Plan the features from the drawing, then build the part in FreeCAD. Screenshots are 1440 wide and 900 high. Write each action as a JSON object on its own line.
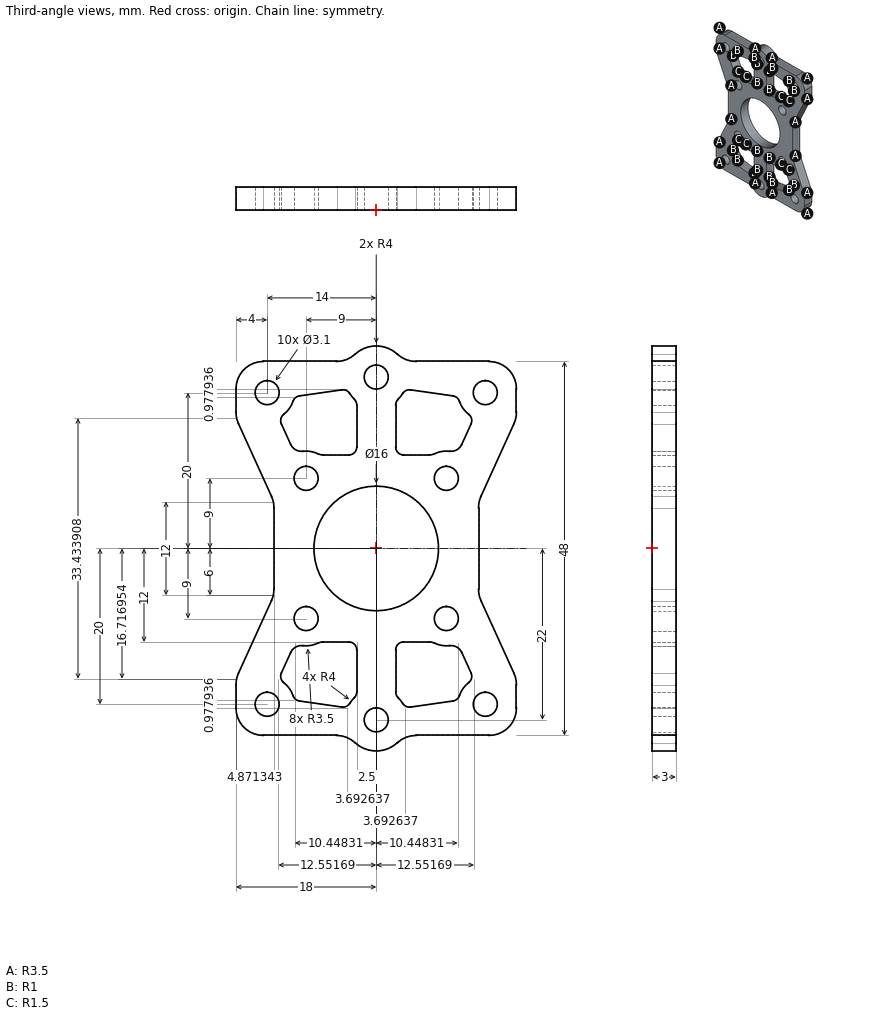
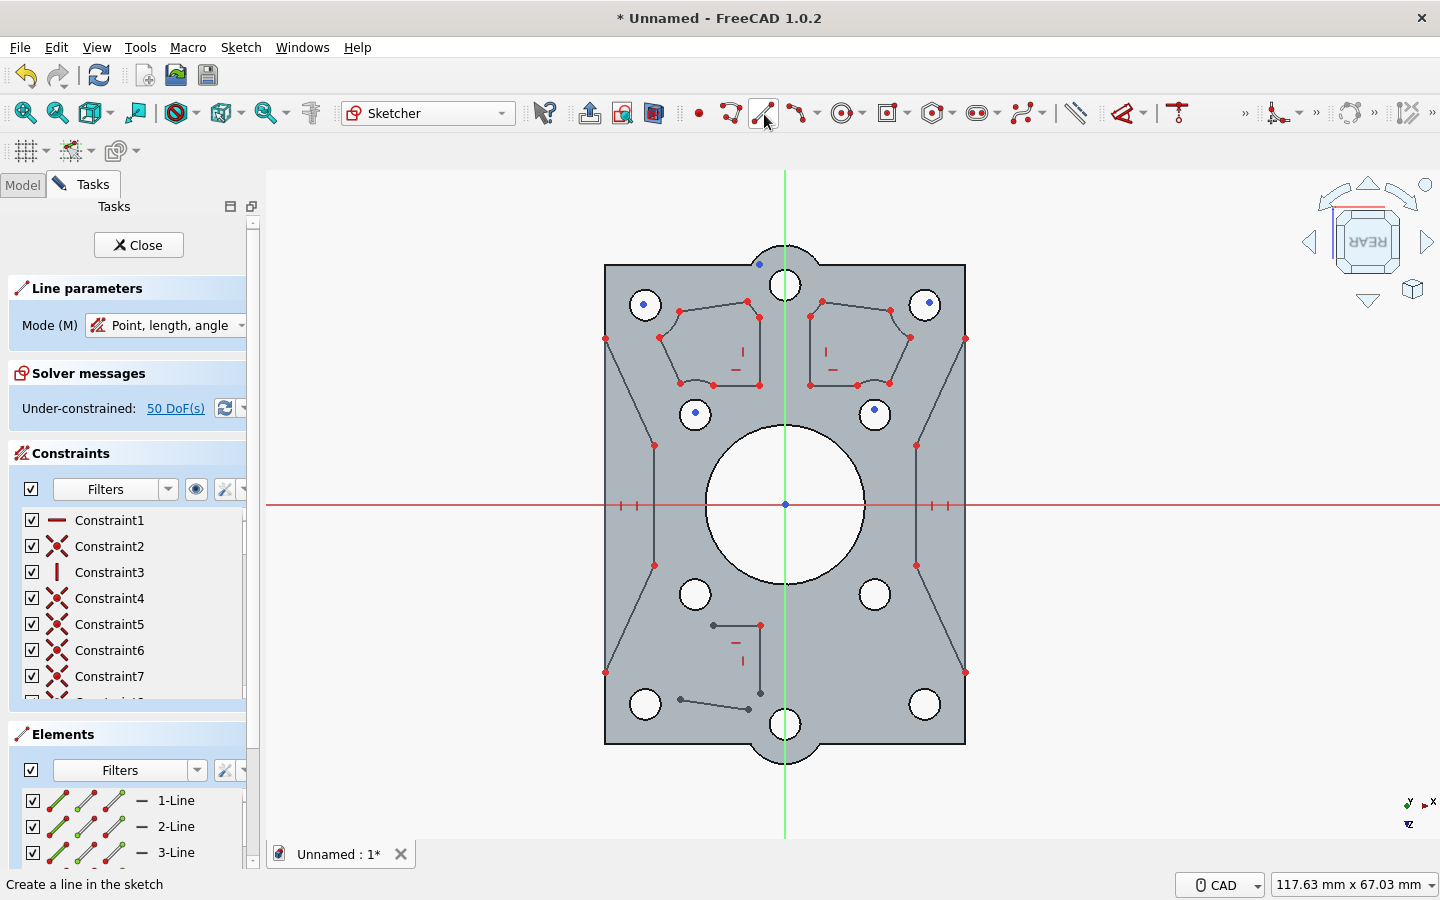
{"action": "left_click", "coordinate": [681, 626]}
{"action": "left_click", "coordinate": [660, 673]}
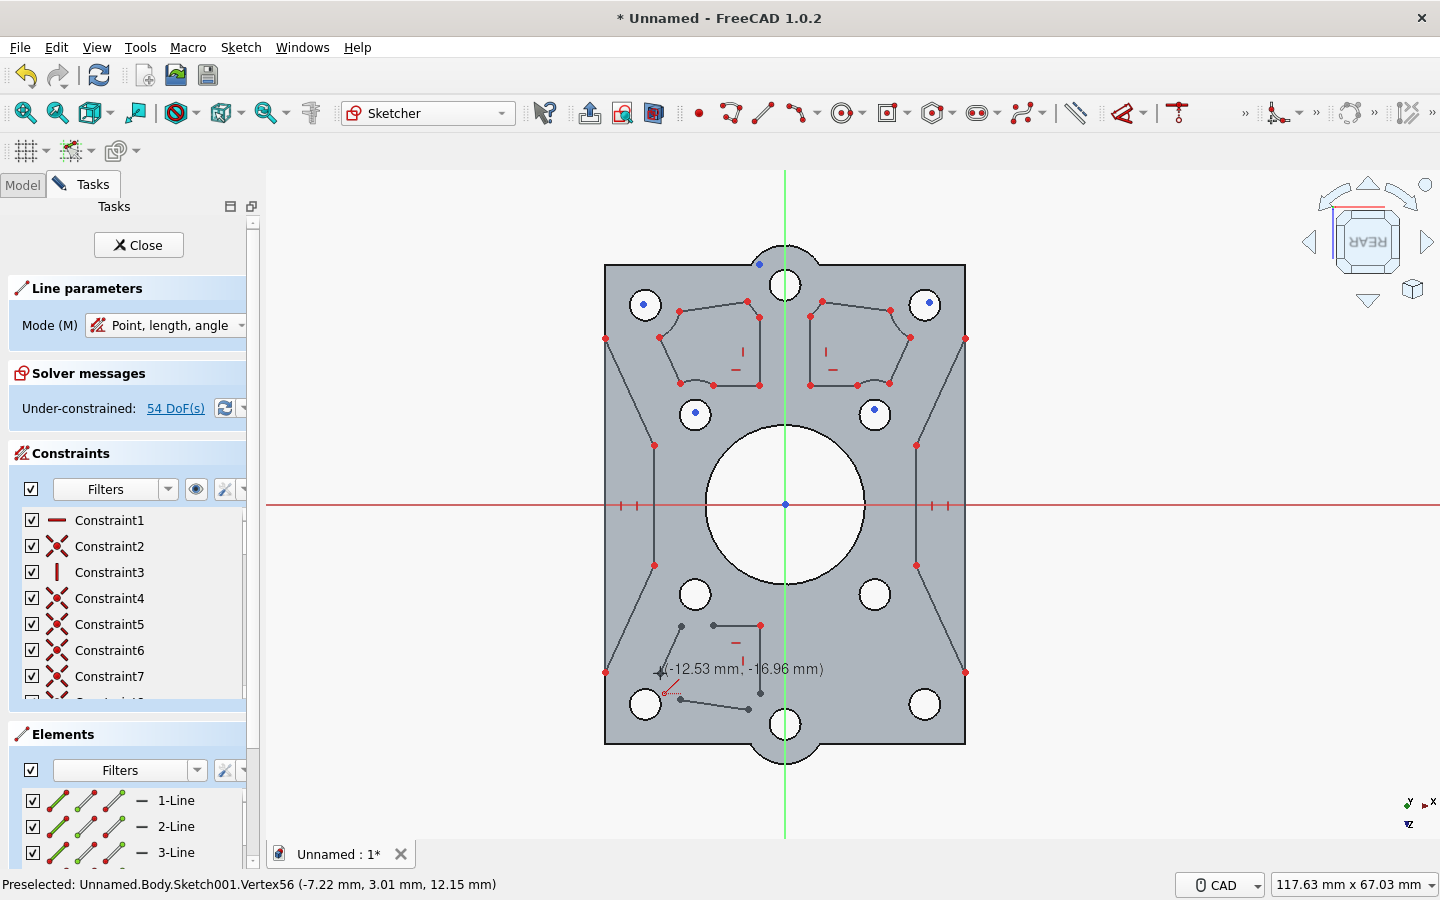
{"action": "left_click", "coordinate": [796, 114]}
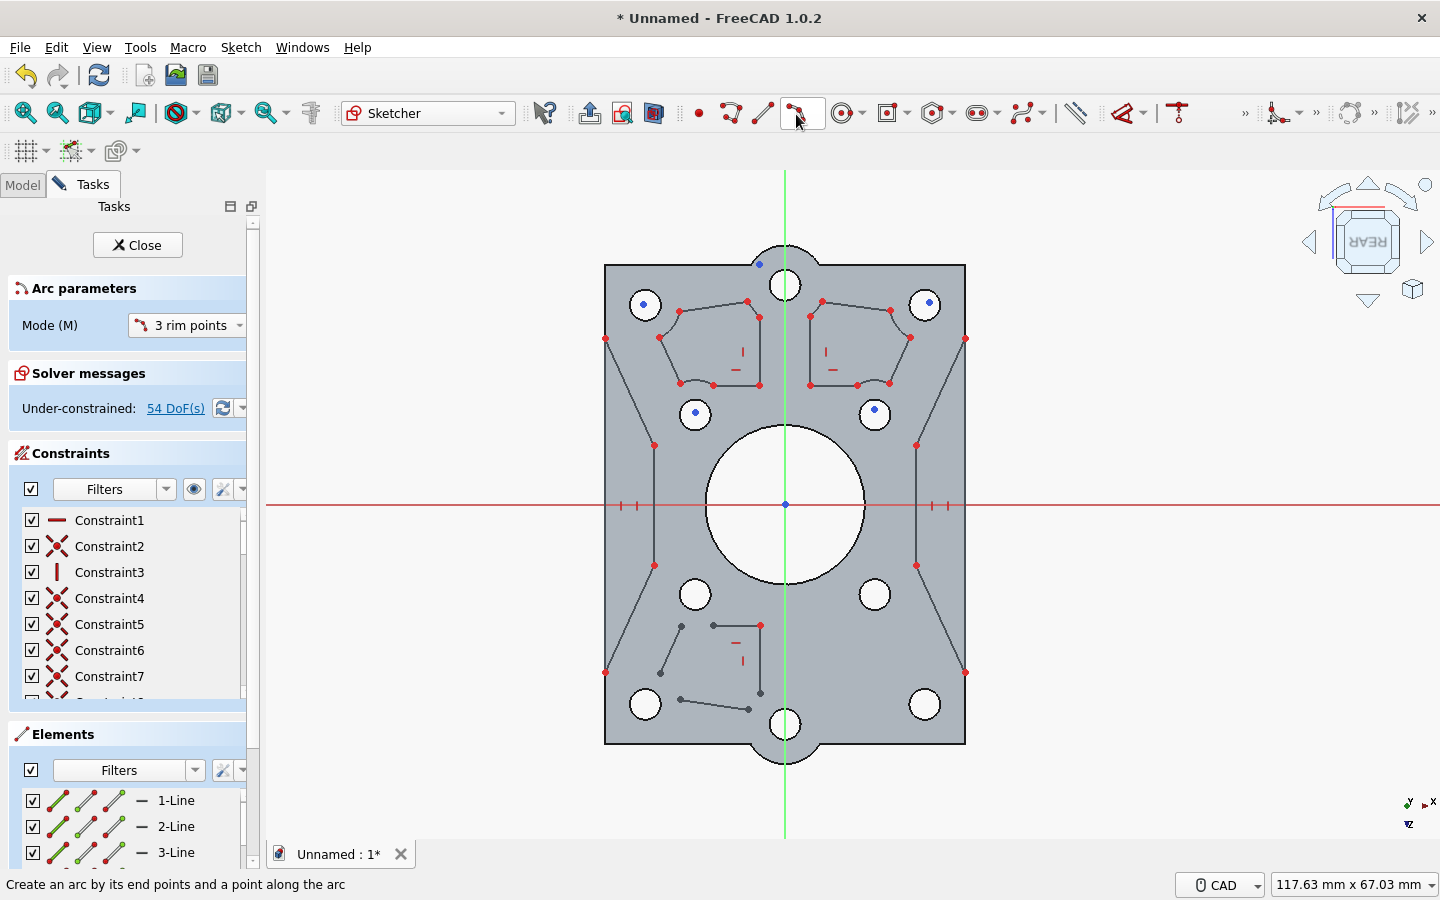
{"action": "left_click", "coordinate": [748, 710]}
{"action": "left_click", "coordinate": [760, 694]}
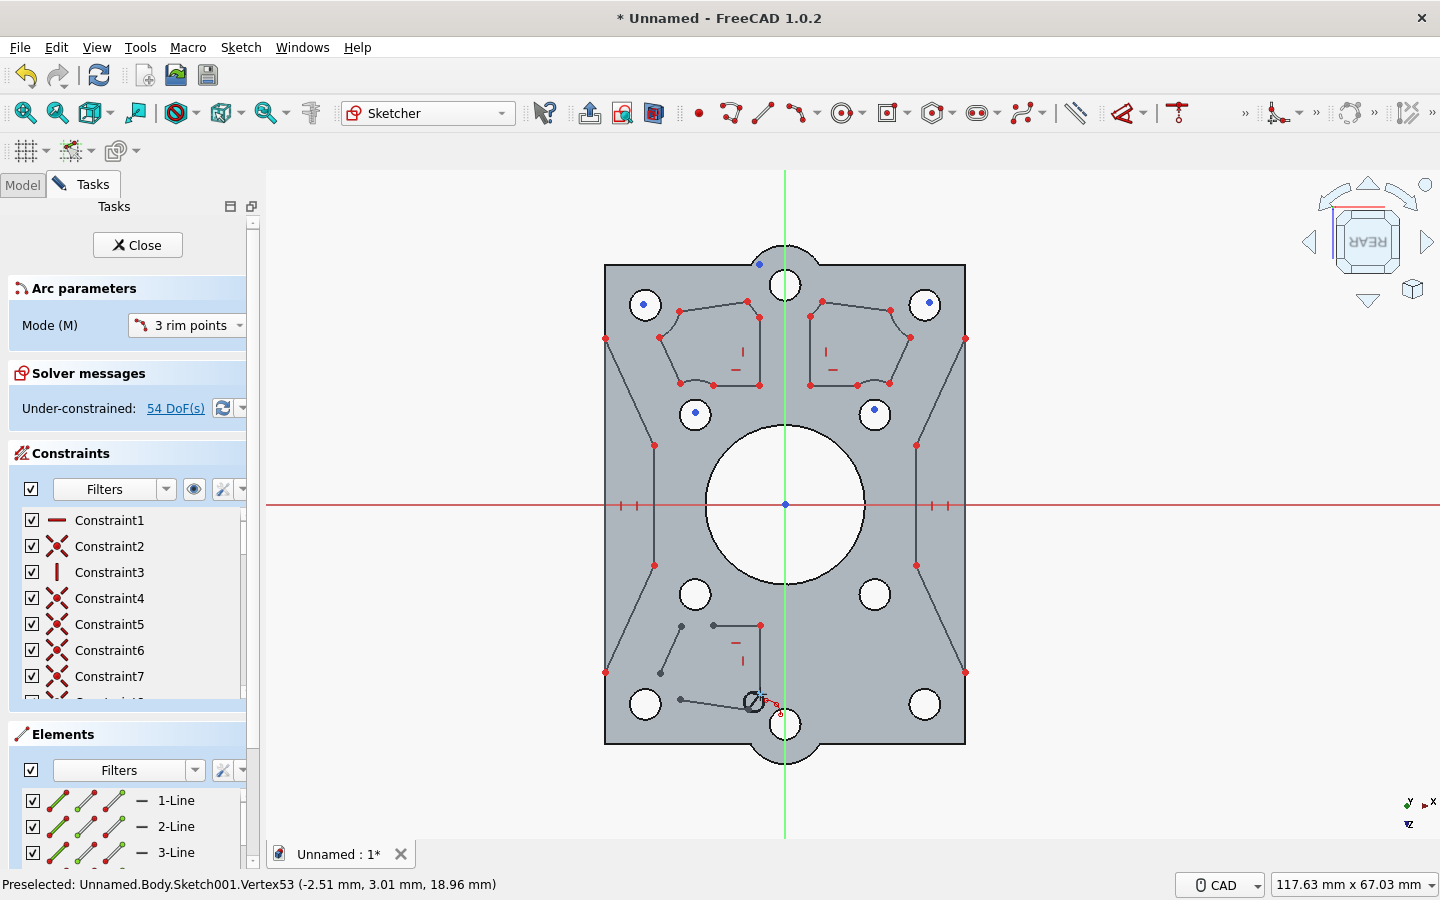
{"action": "scroll", "coordinate": [753, 700], "scroll_direction": "up", "scroll_amount": 13}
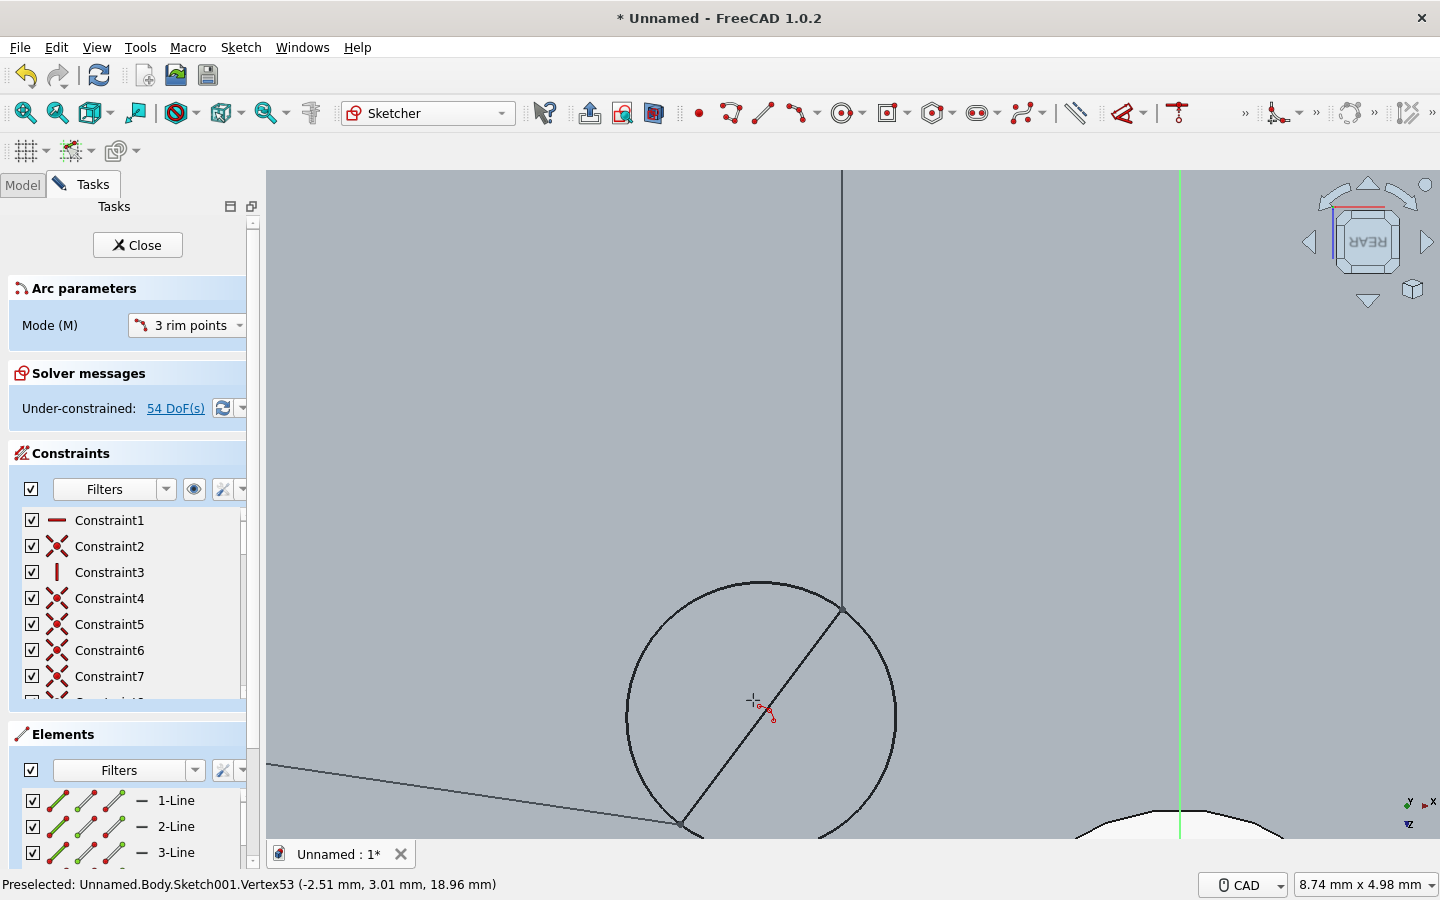
{"action": "left_click", "coordinate": [750, 694]}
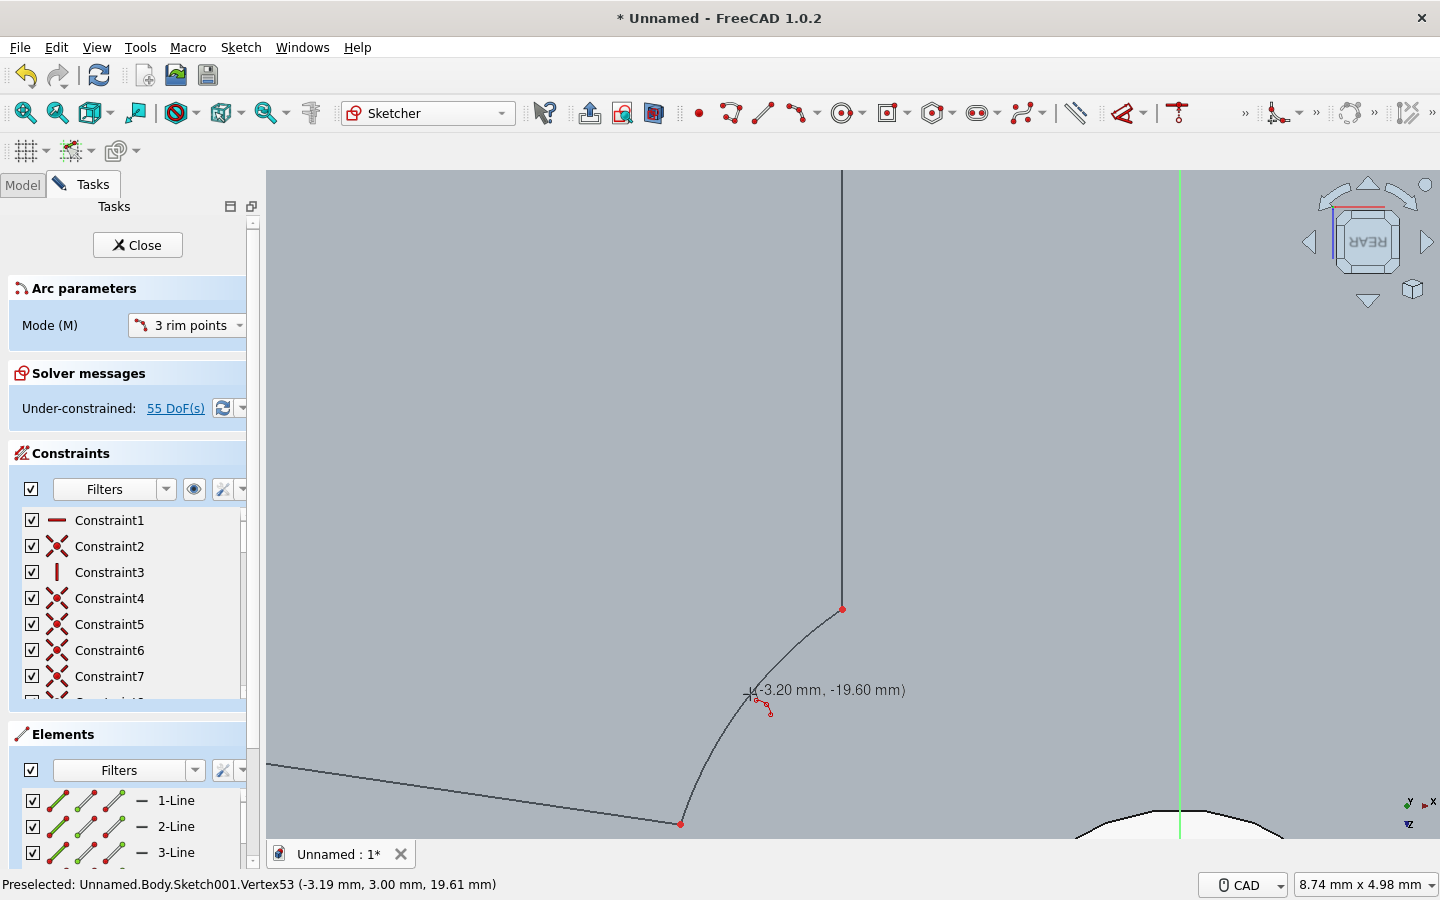
{"action": "scroll", "coordinate": [753, 701], "scroll_direction": "down", "scroll_amount": 13}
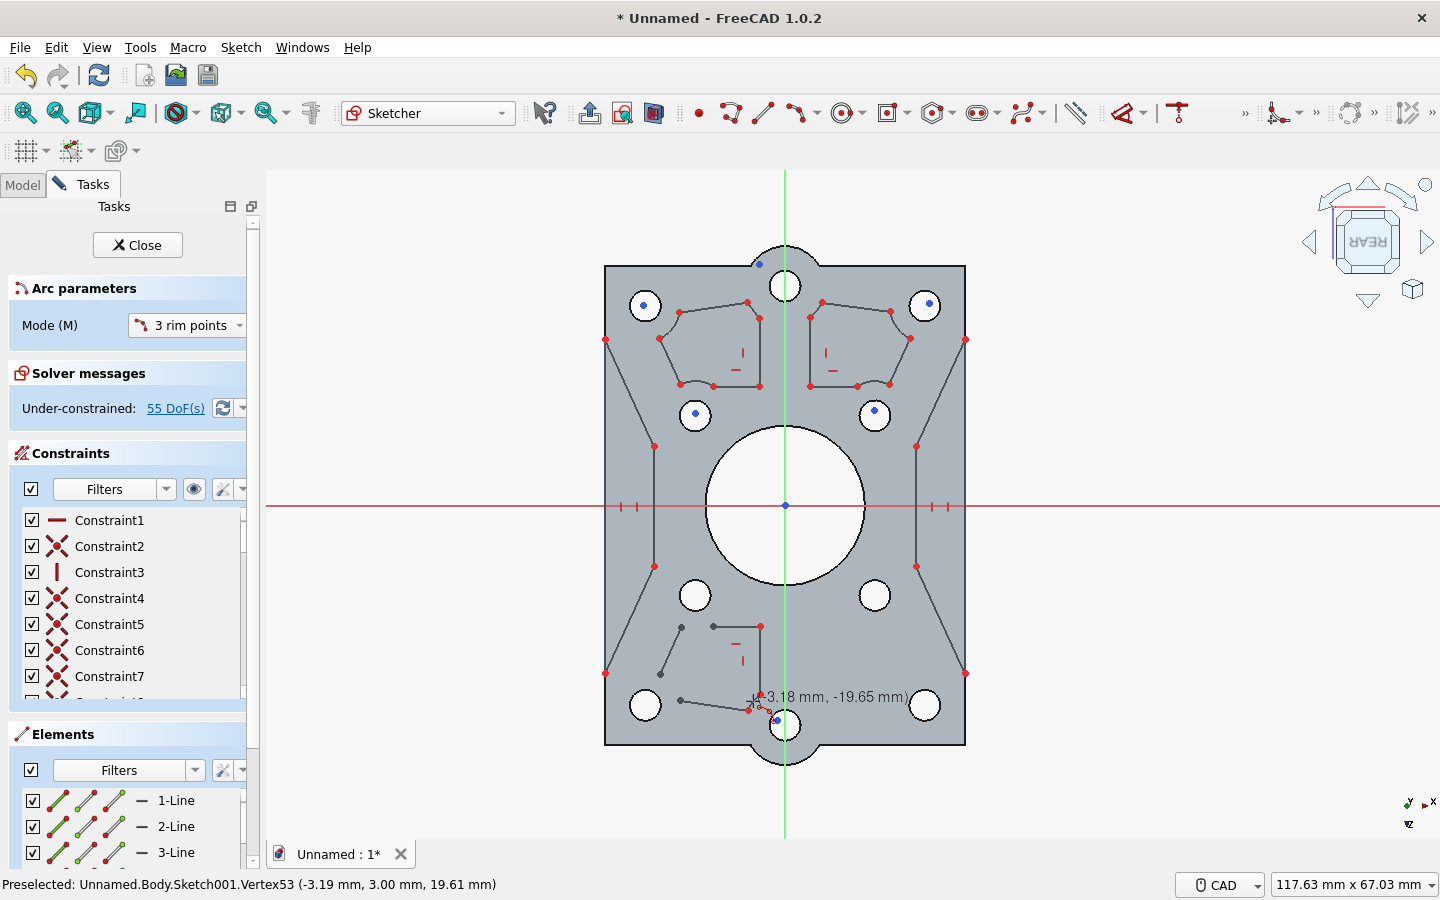
{"action": "left_click", "coordinate": [713, 627]}
{"action": "left_click", "coordinate": [681, 628]}